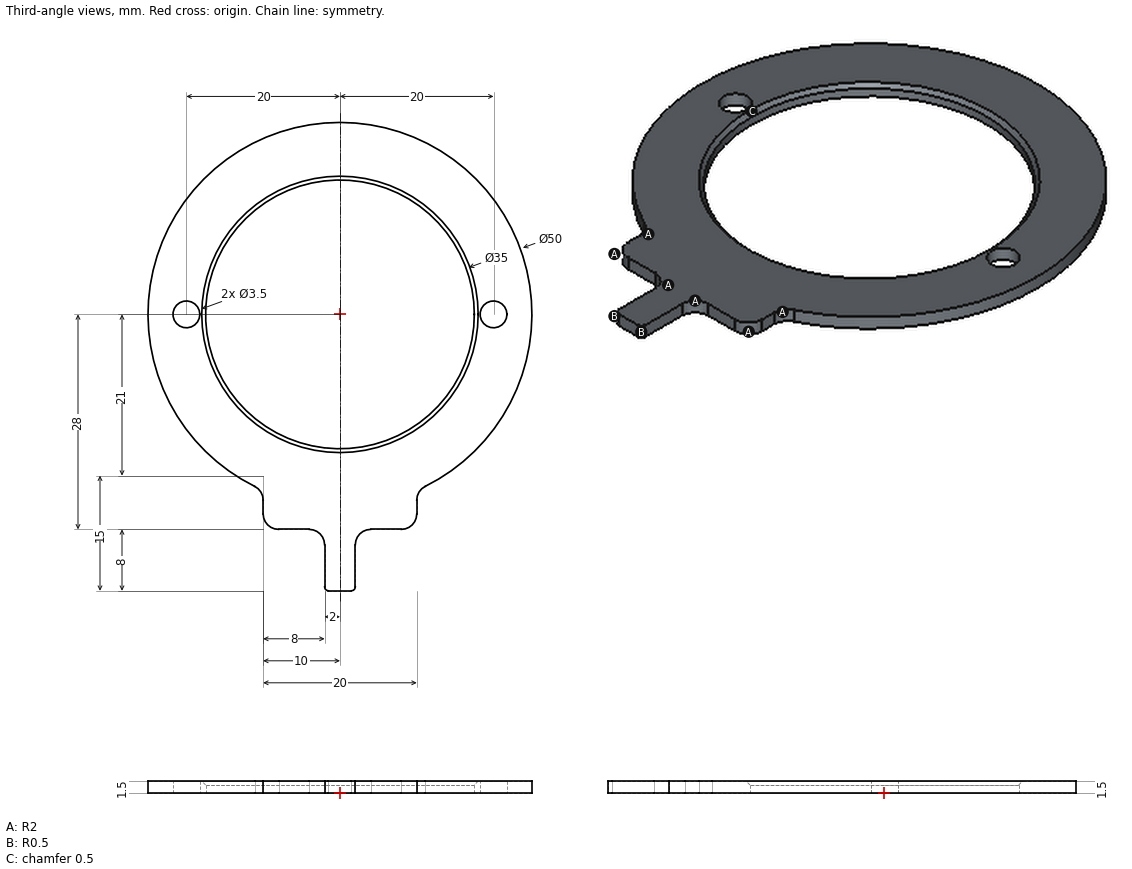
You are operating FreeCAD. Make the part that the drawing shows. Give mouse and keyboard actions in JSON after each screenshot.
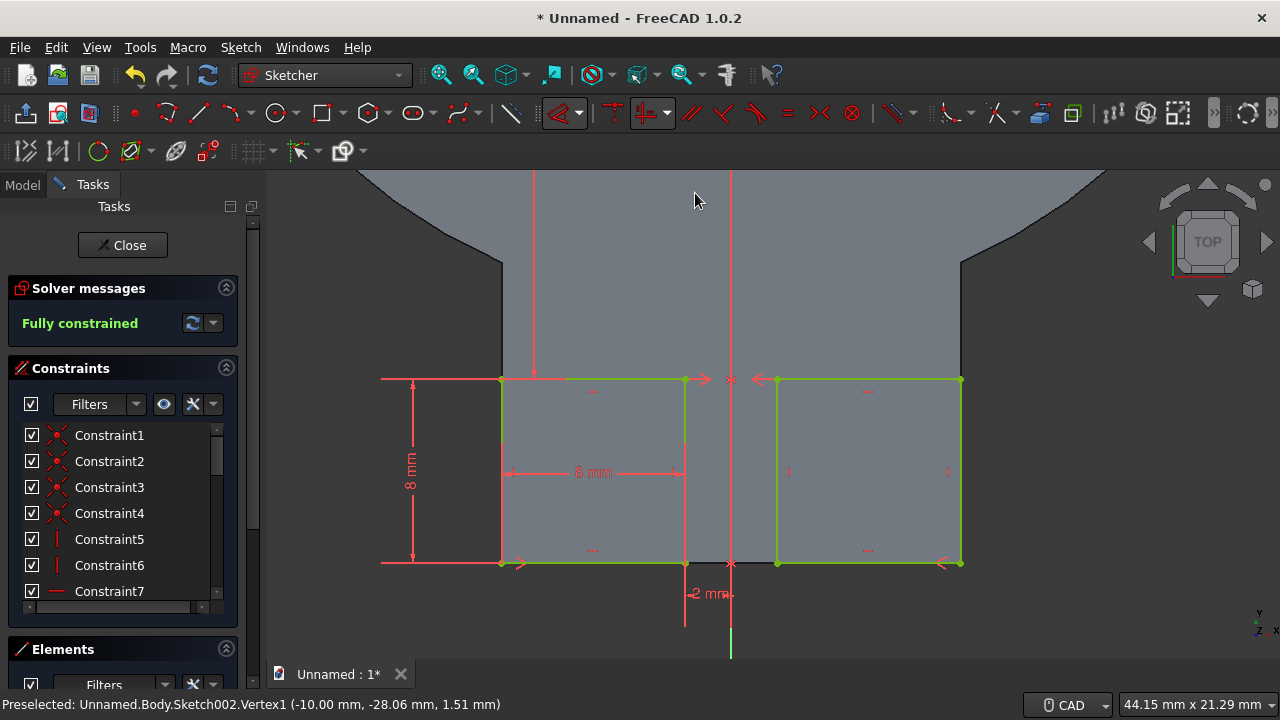
{"action": "left_click", "coordinate": [123, 245]}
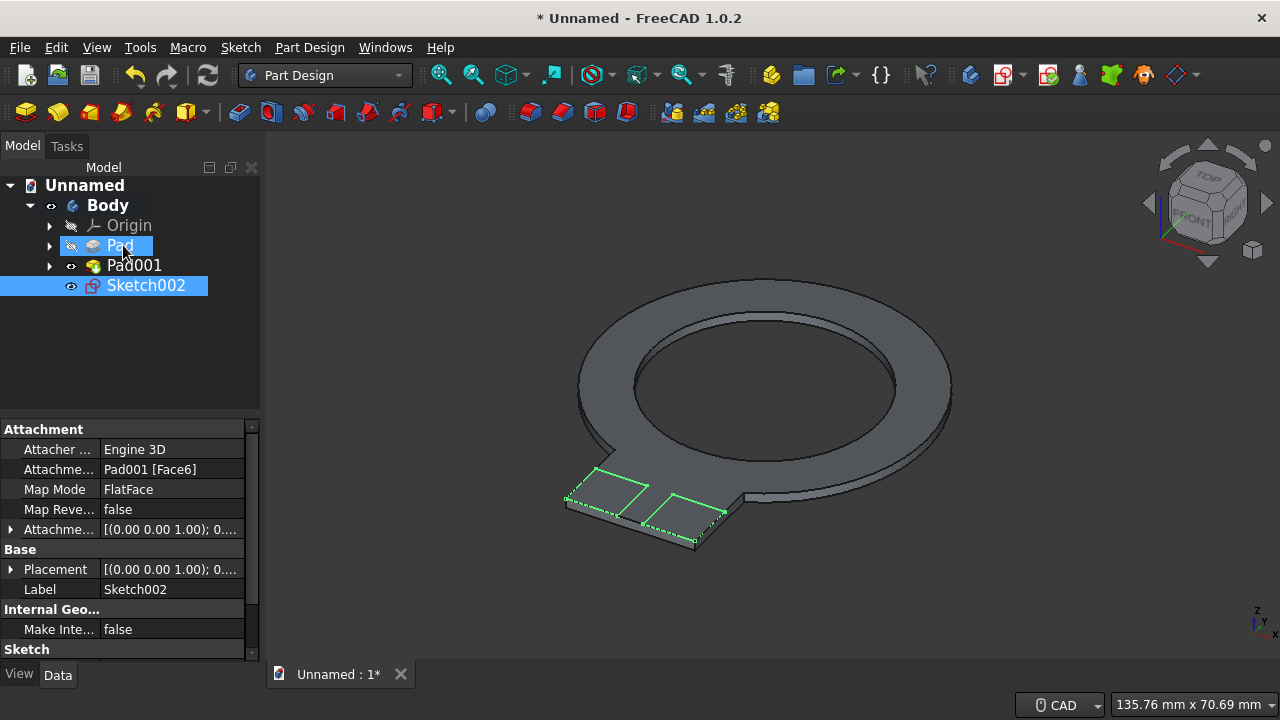
{"action": "left_click", "coordinate": [240, 112]}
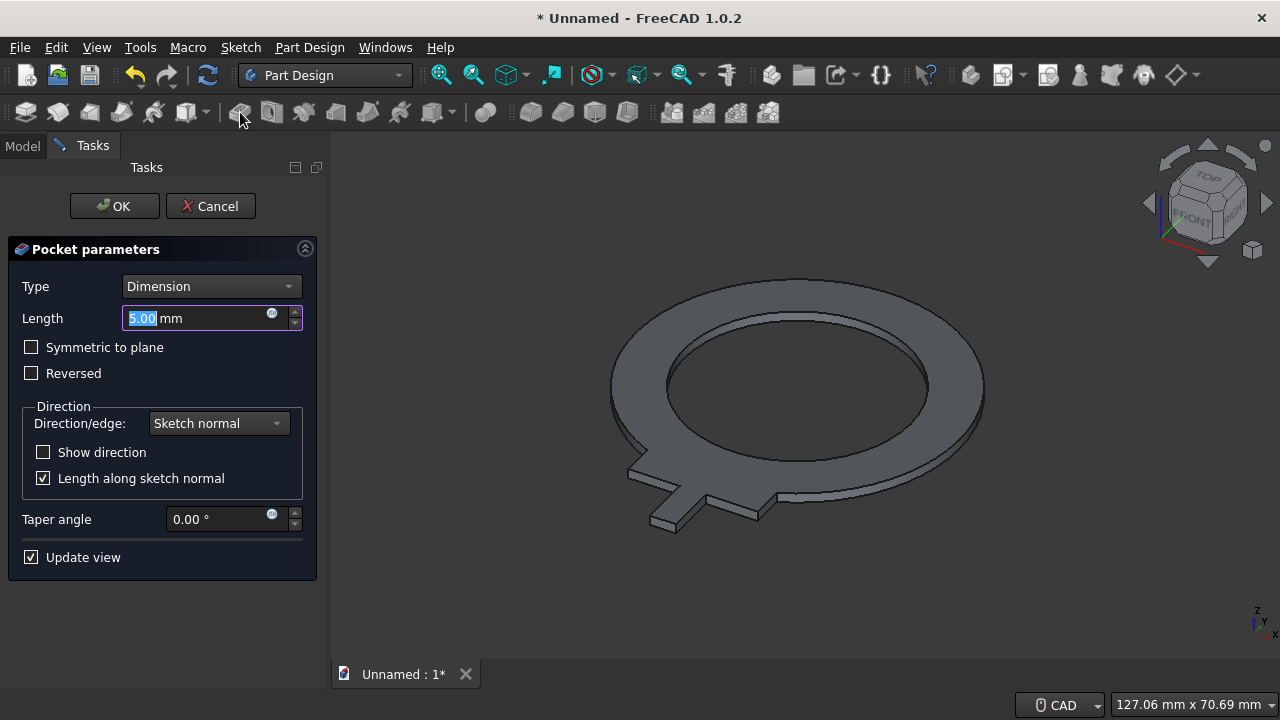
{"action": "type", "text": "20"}
{"action": "key", "text": "Tab"}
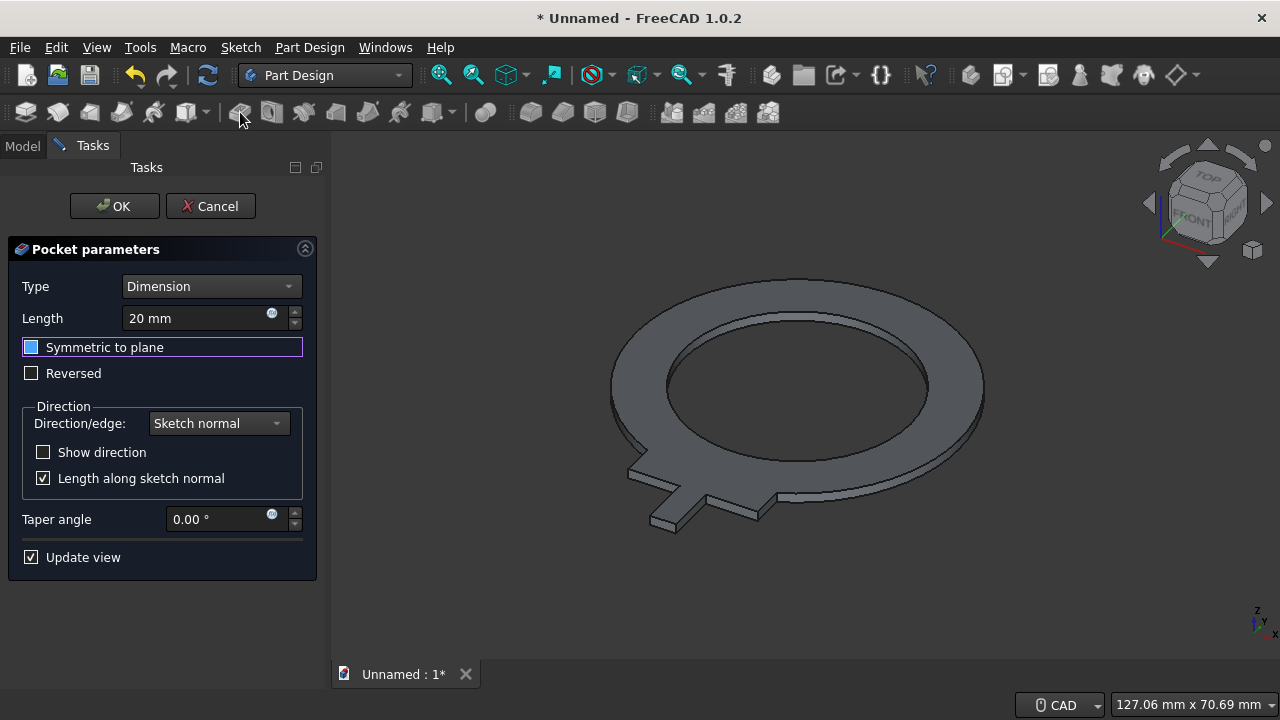
{"action": "left_click", "coordinate": [115, 206]}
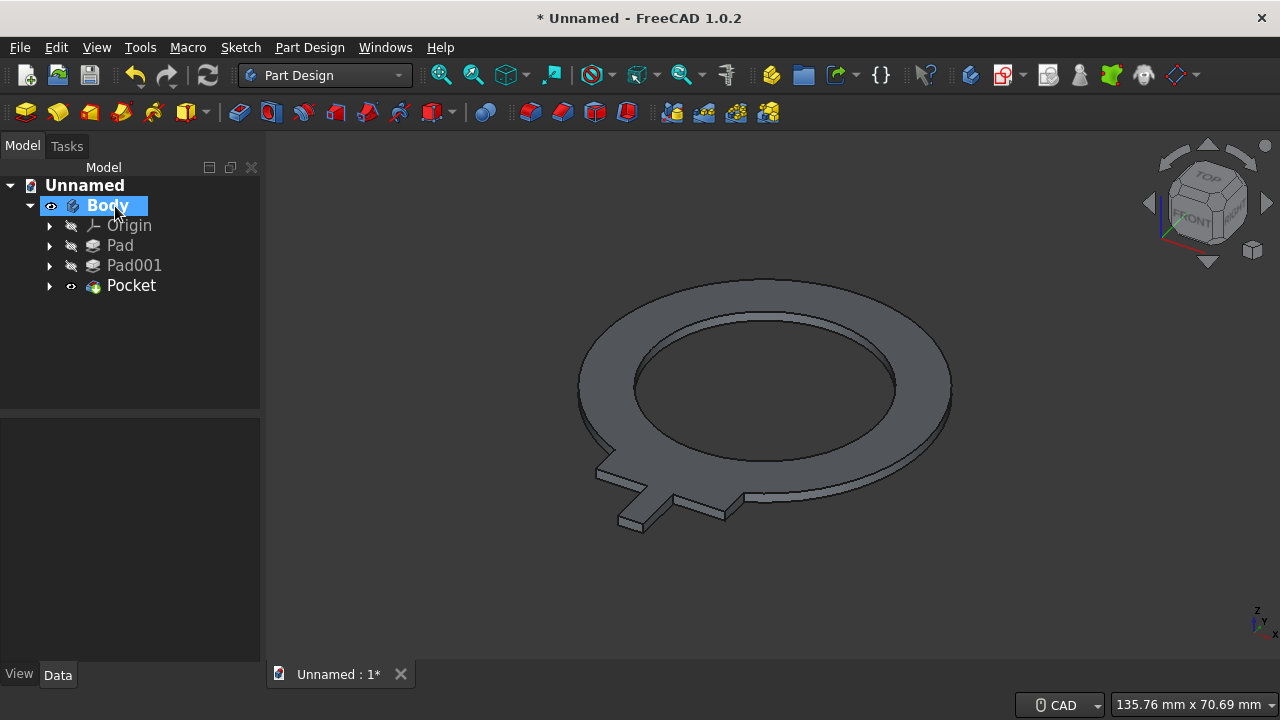
{"action": "left_click", "coordinate": [725, 517]}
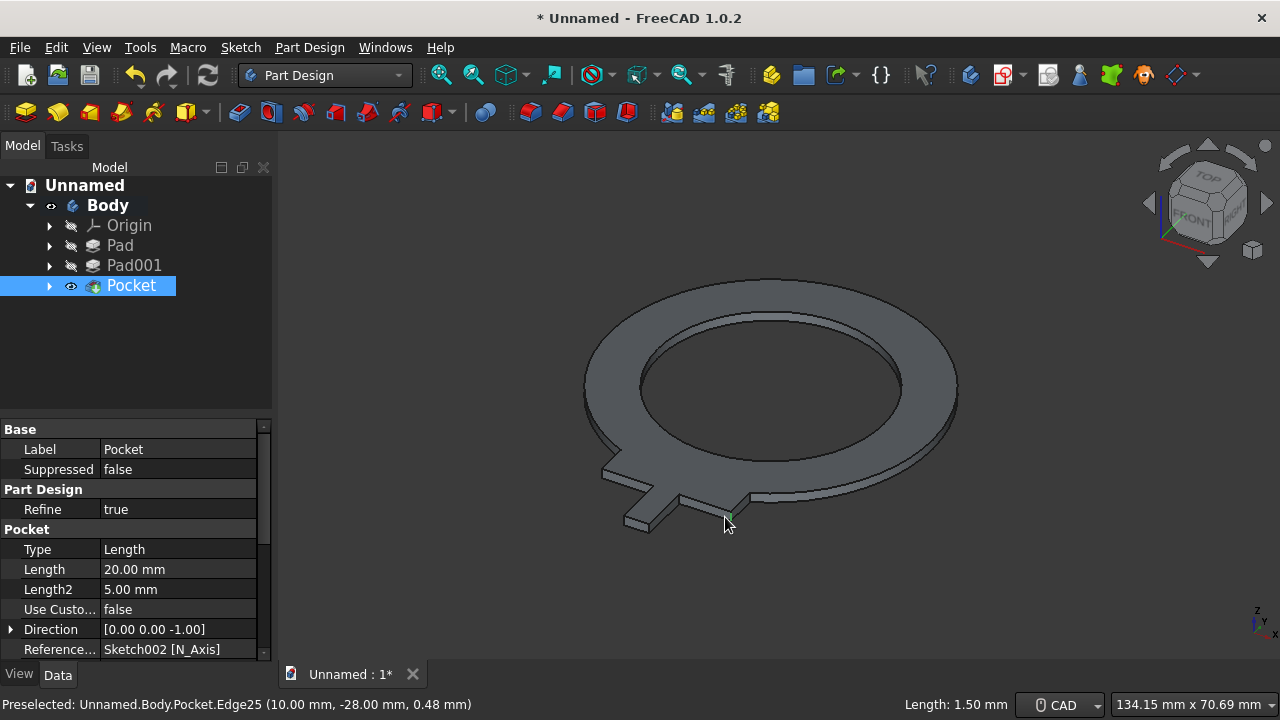
{"action": "scroll", "coordinate": [750, 496], "scroll_direction": "up", "scroll_amount": 7}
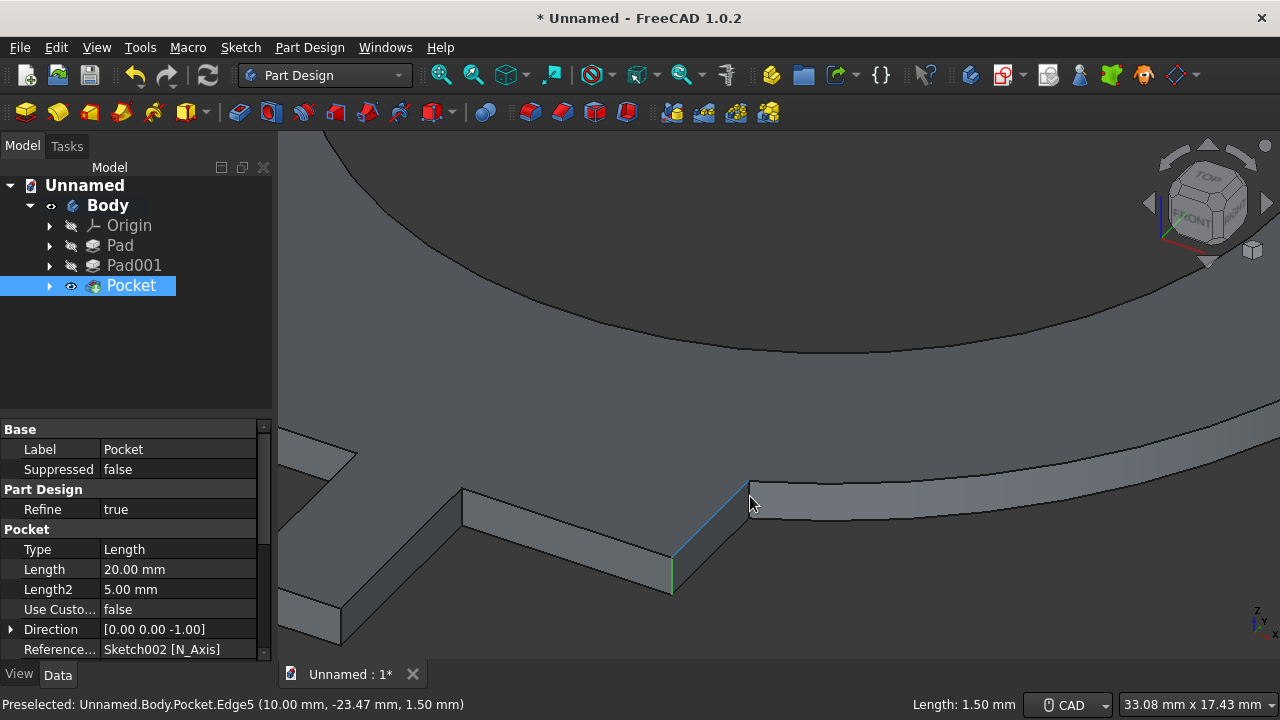
{"action": "left_click", "coordinate": [442, 76]}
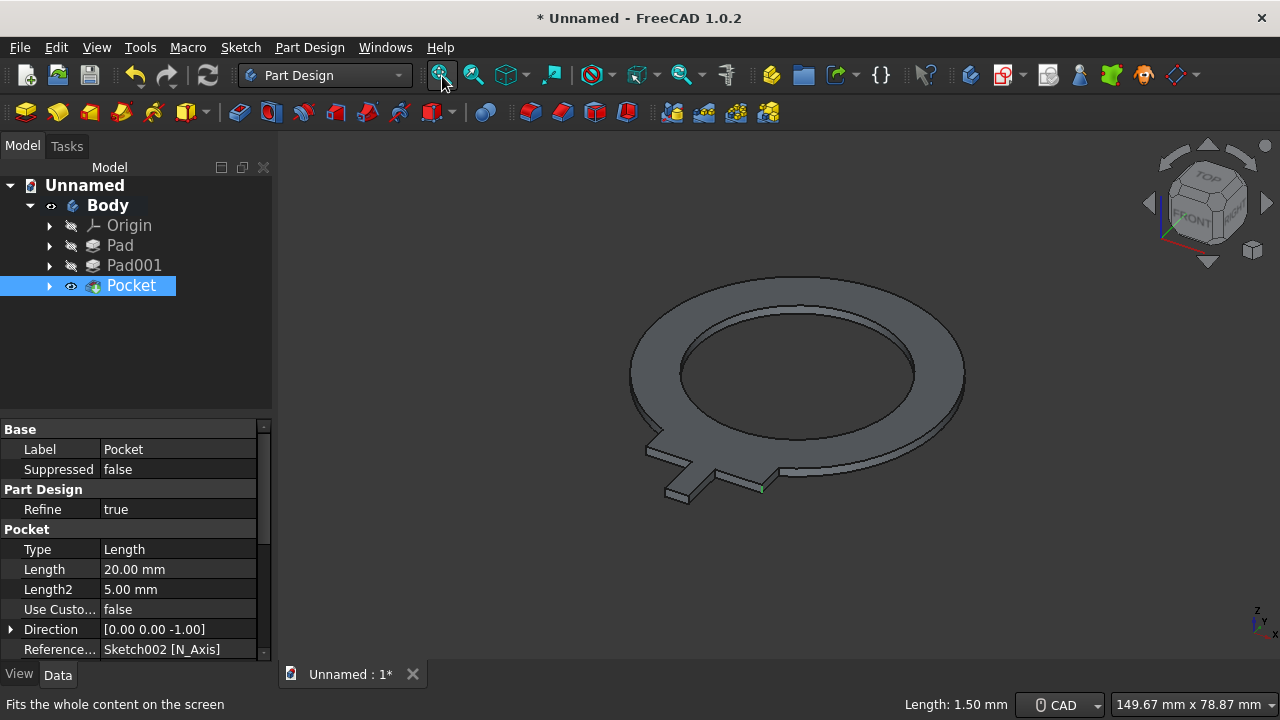
{"action": "key", "text": "0"}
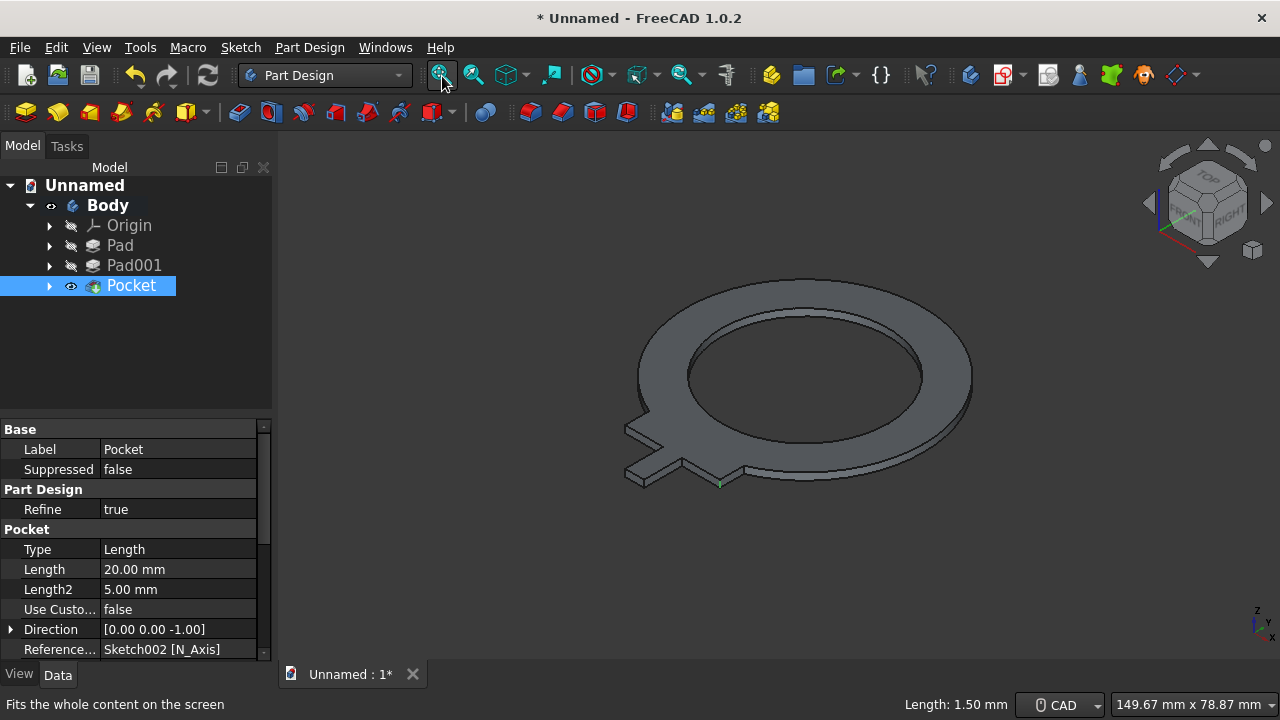
{"action": "scroll", "coordinate": [744, 469], "scroll_direction": "up", "scroll_amount": 7}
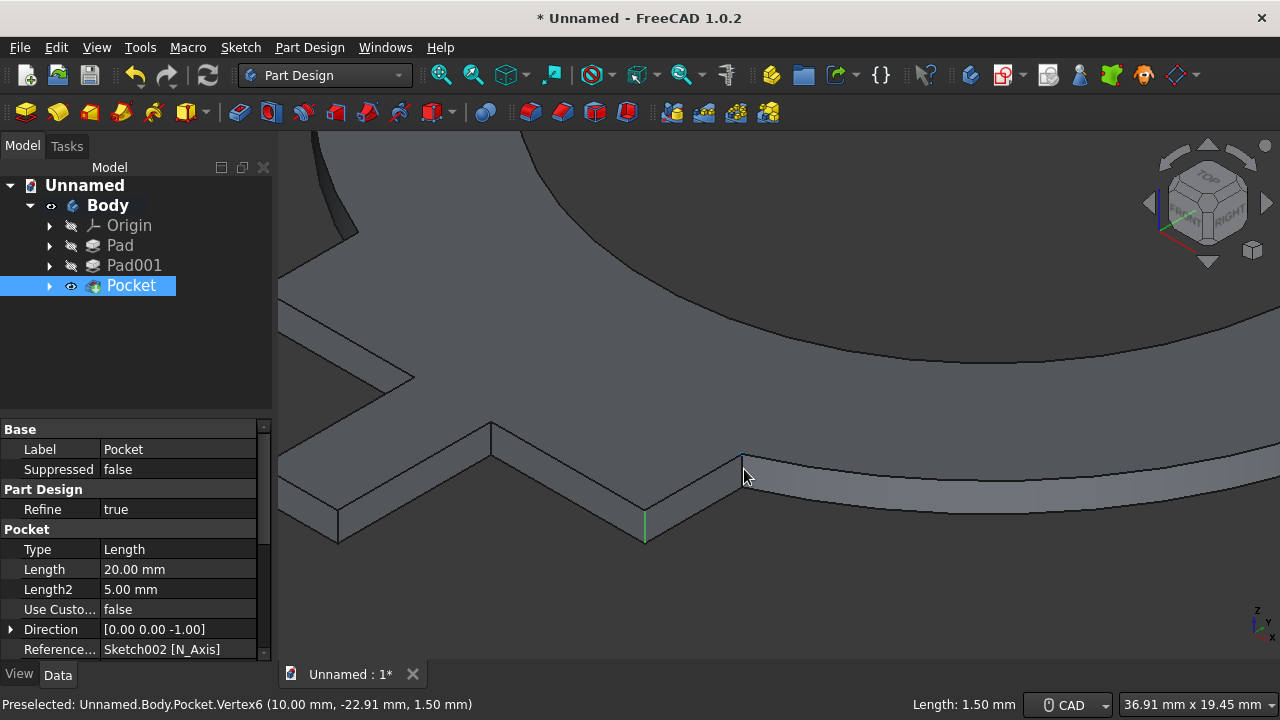
{"action": "left_click", "coordinate": [442, 76]}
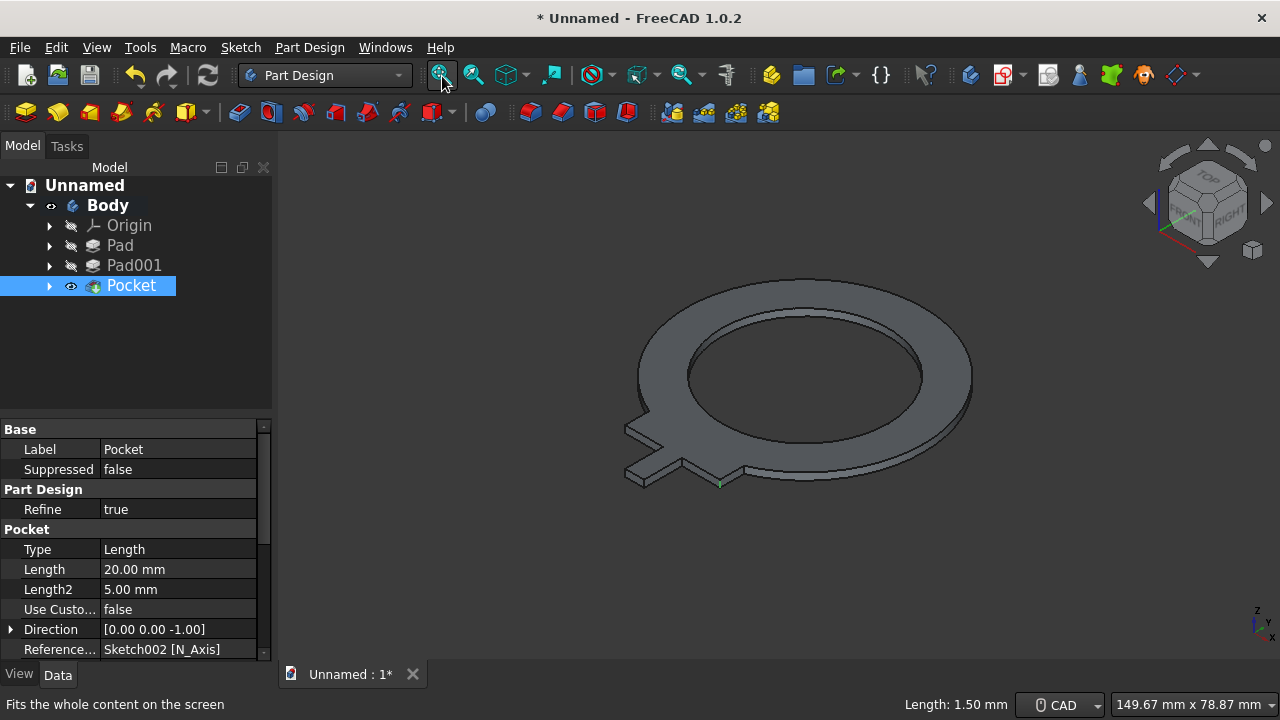
{"action": "key", "text": "2"}